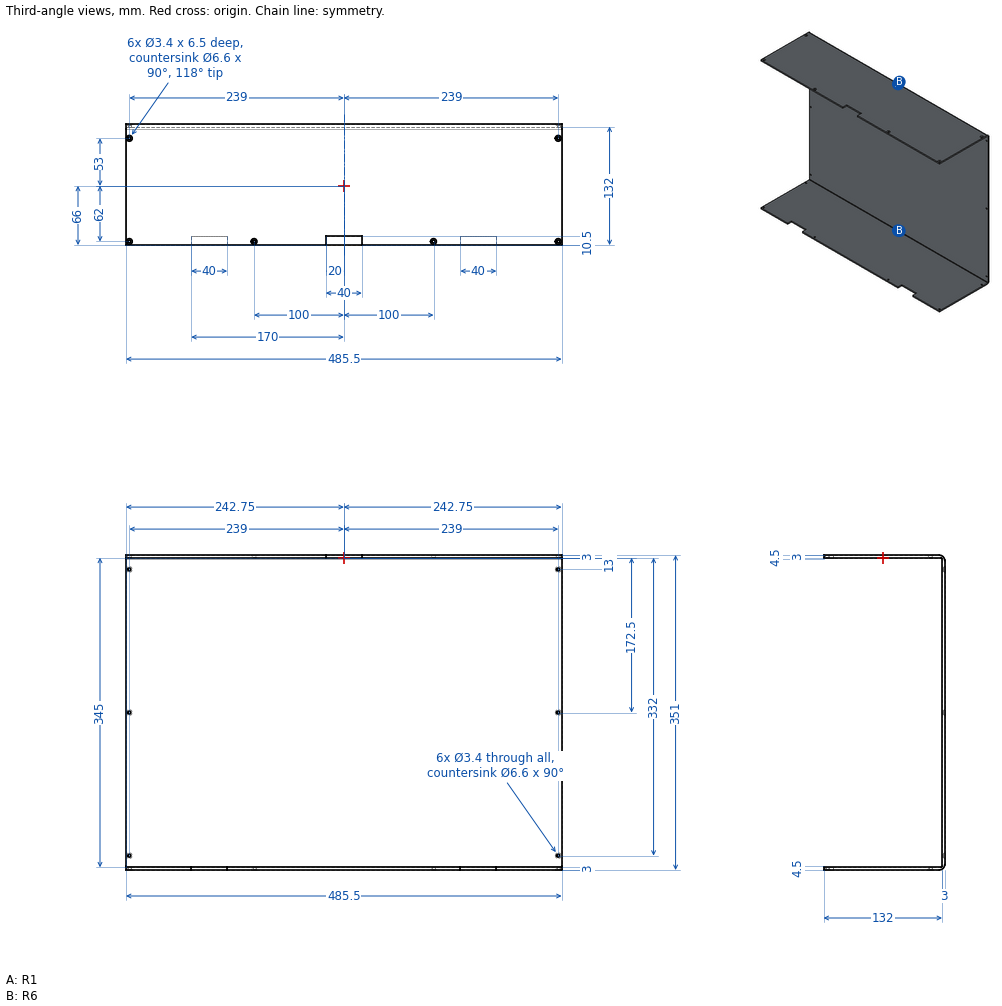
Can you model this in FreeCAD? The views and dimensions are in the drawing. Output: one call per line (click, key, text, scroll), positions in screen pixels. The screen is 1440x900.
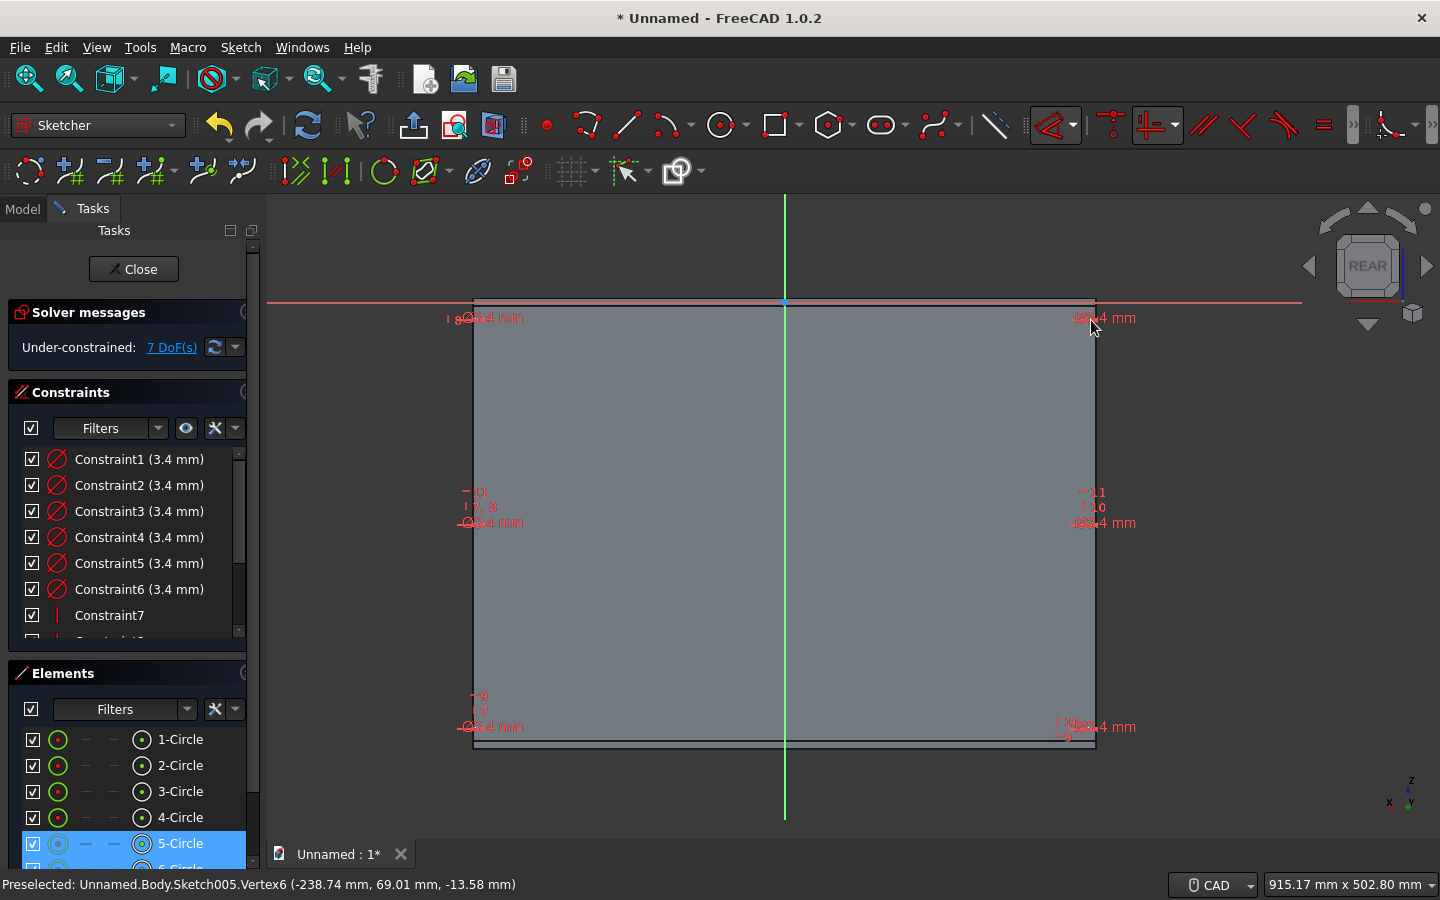
click(1178, 126)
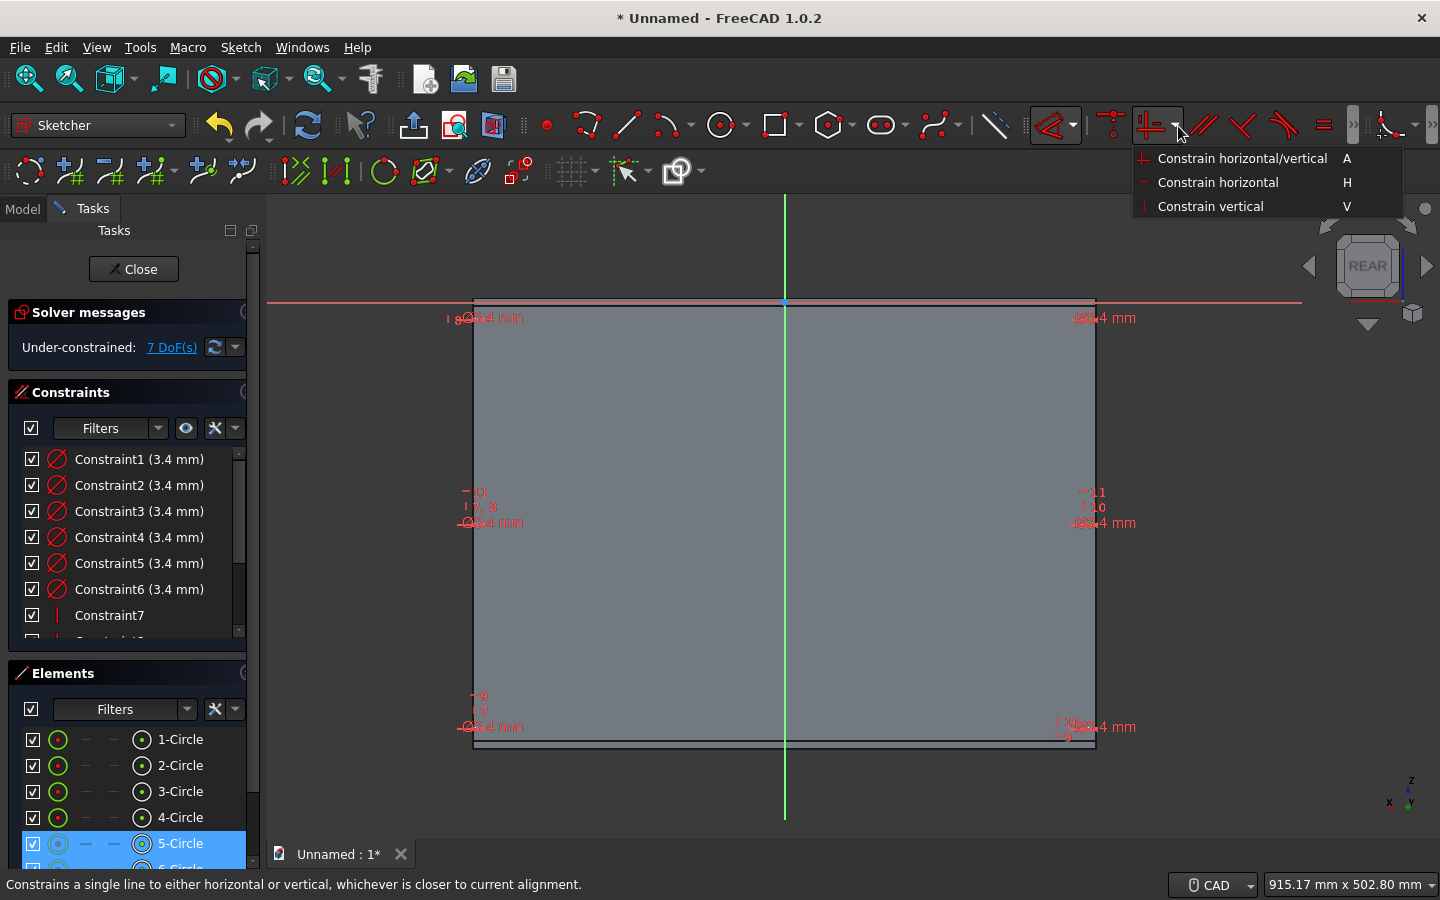
click(1268, 206)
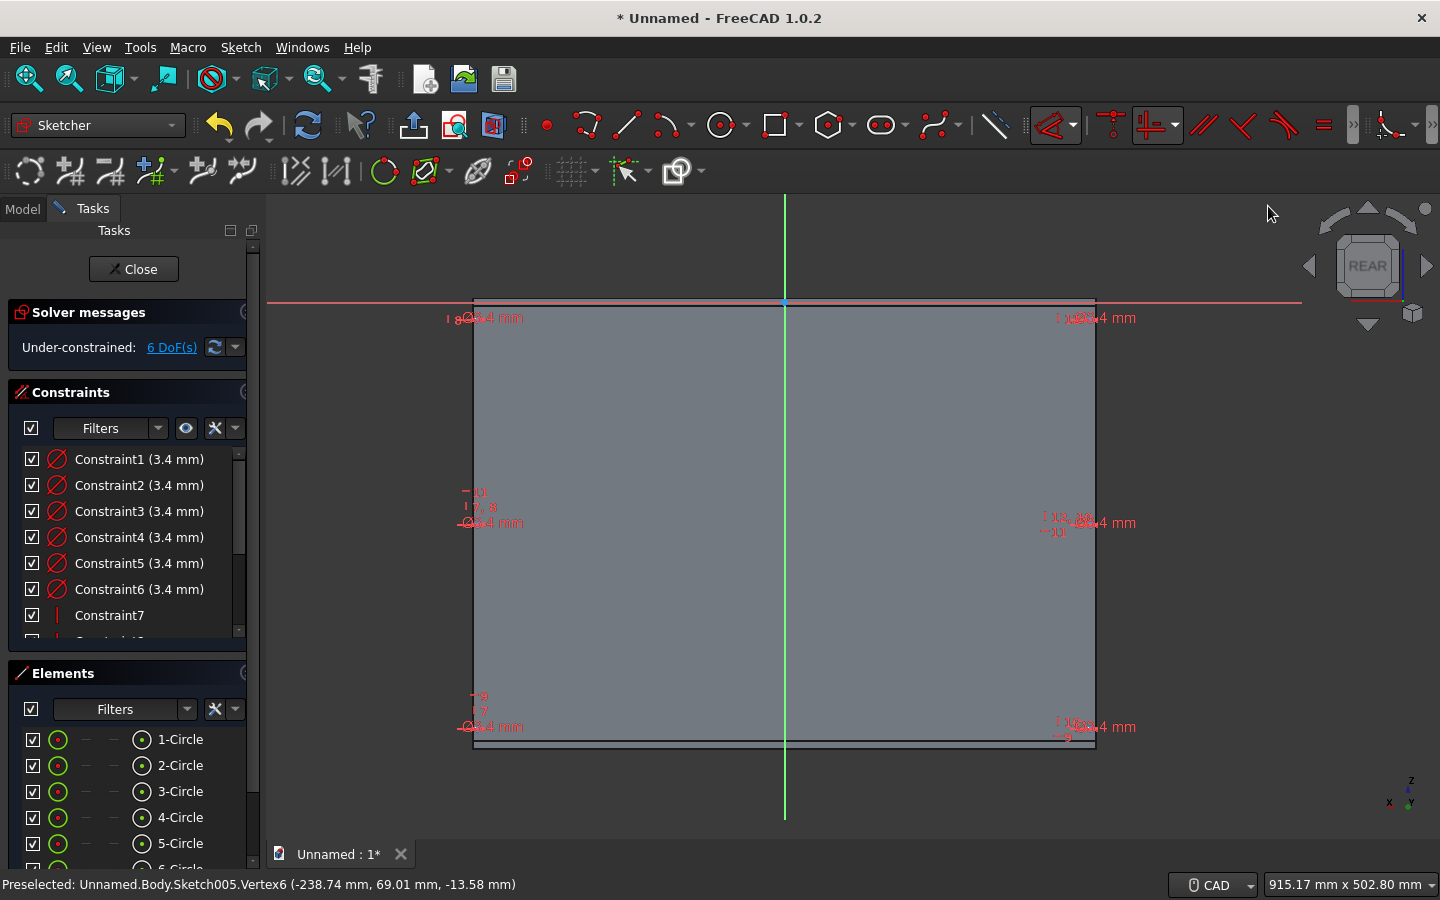
click(478, 320)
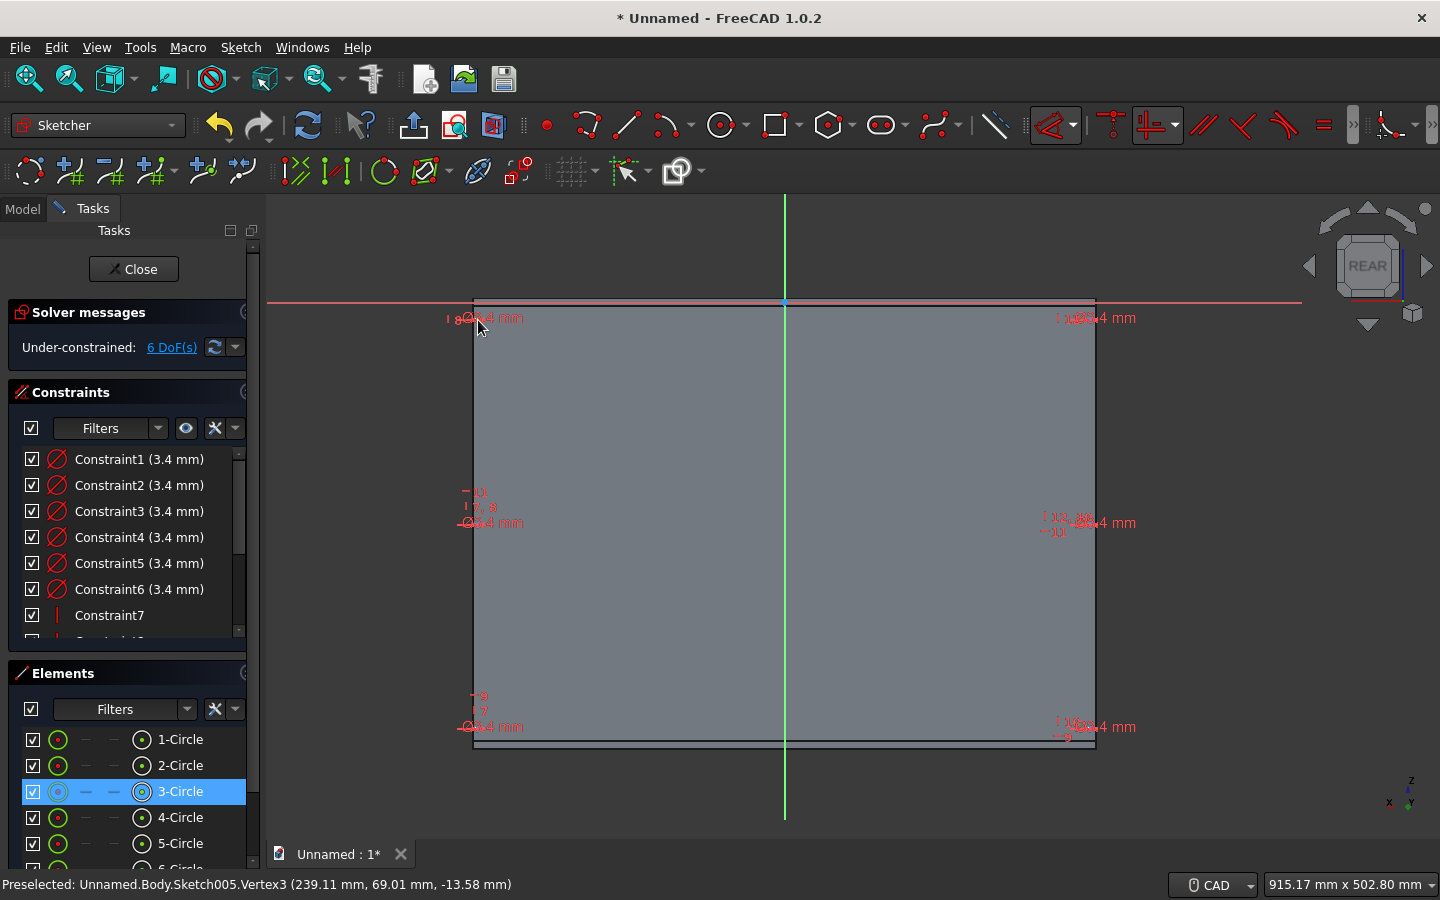
click(1091, 320)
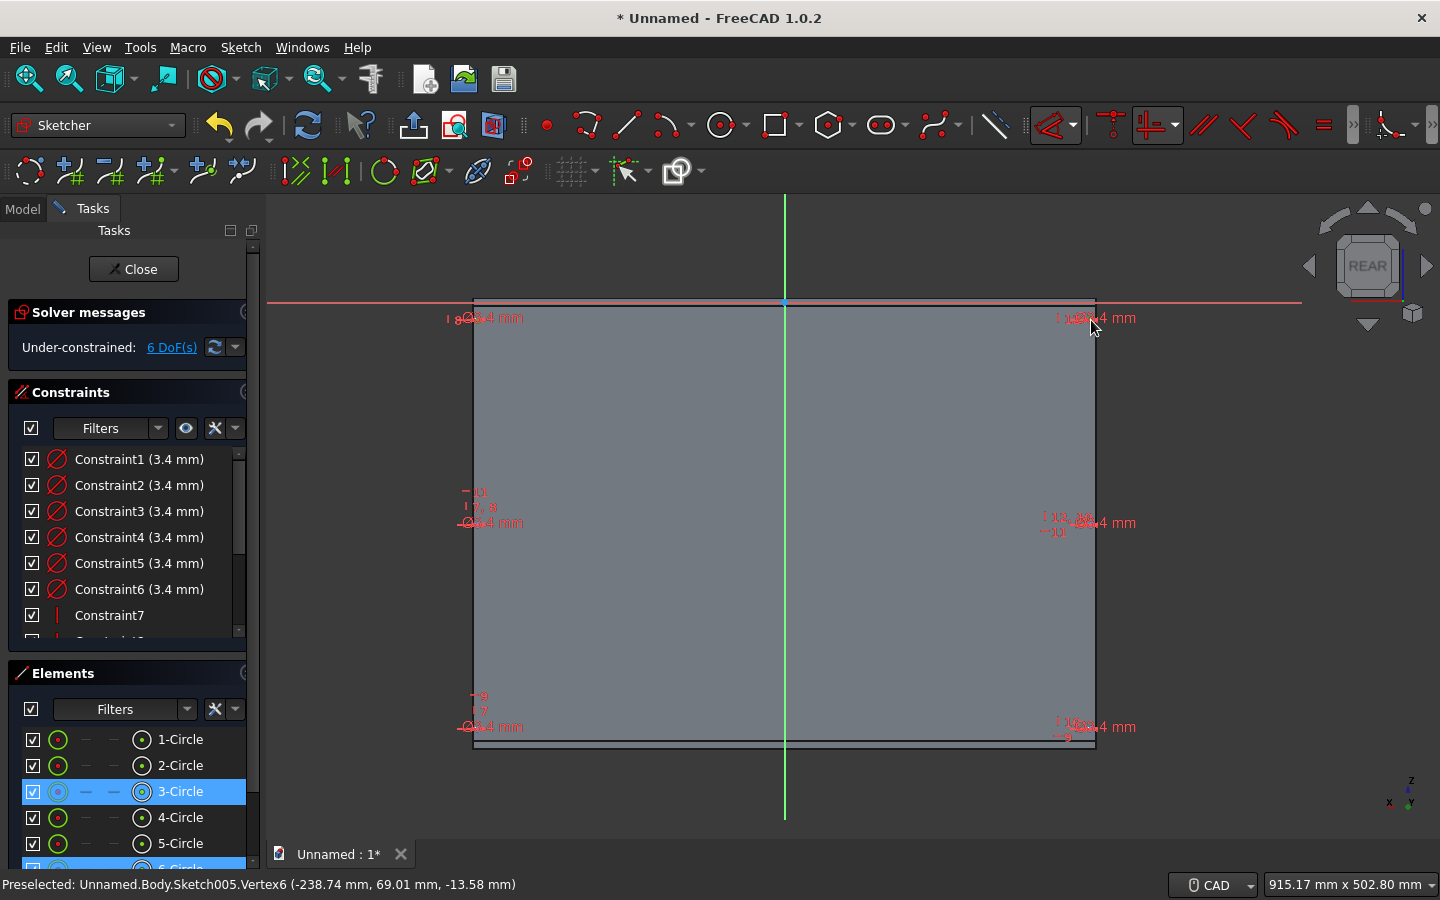
key(h)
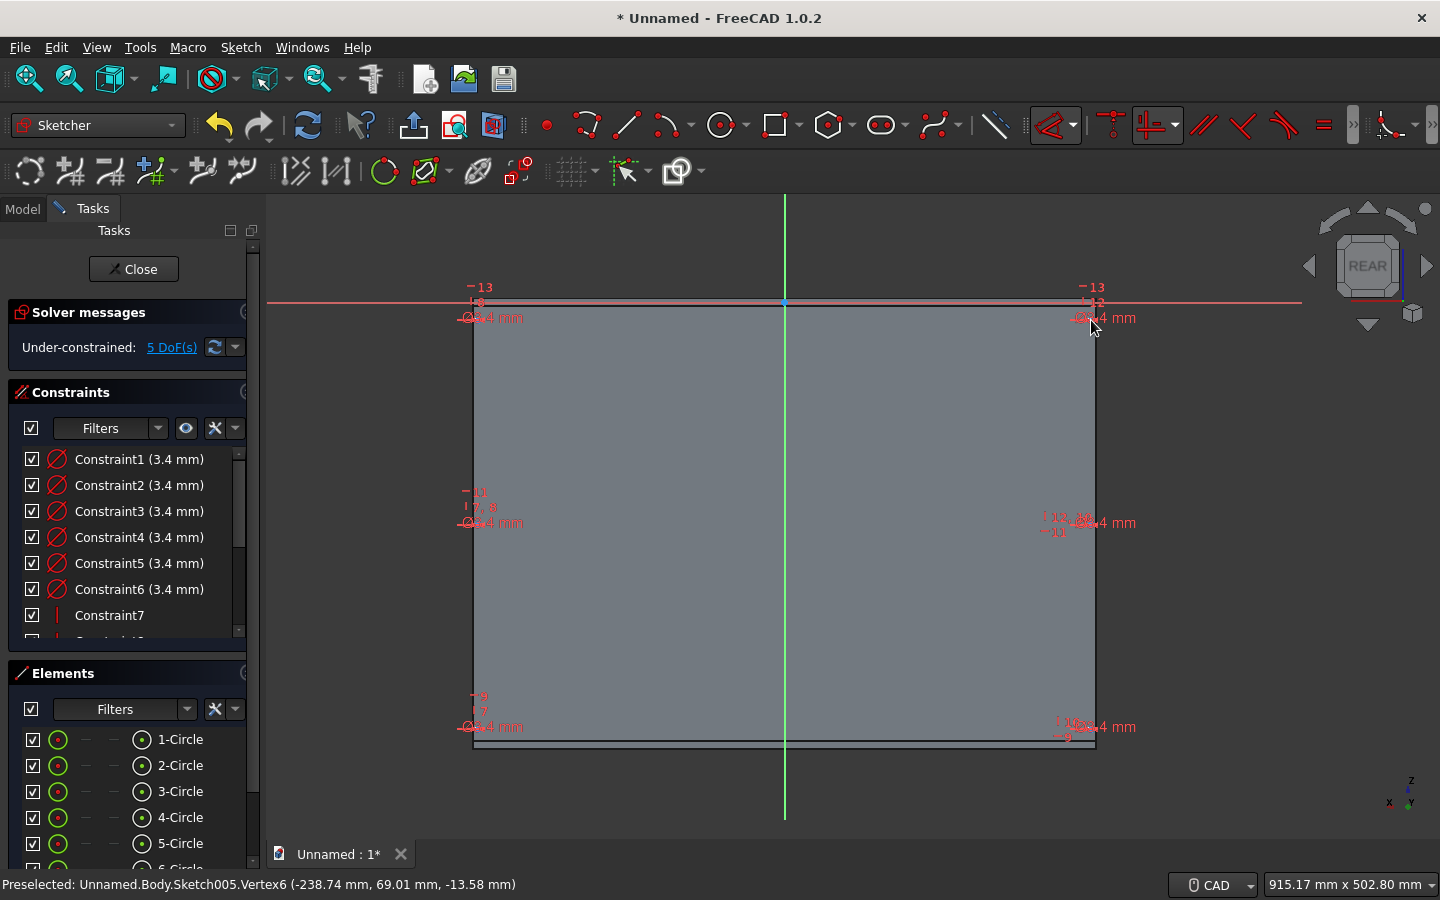
scroll(478, 320, up, 5)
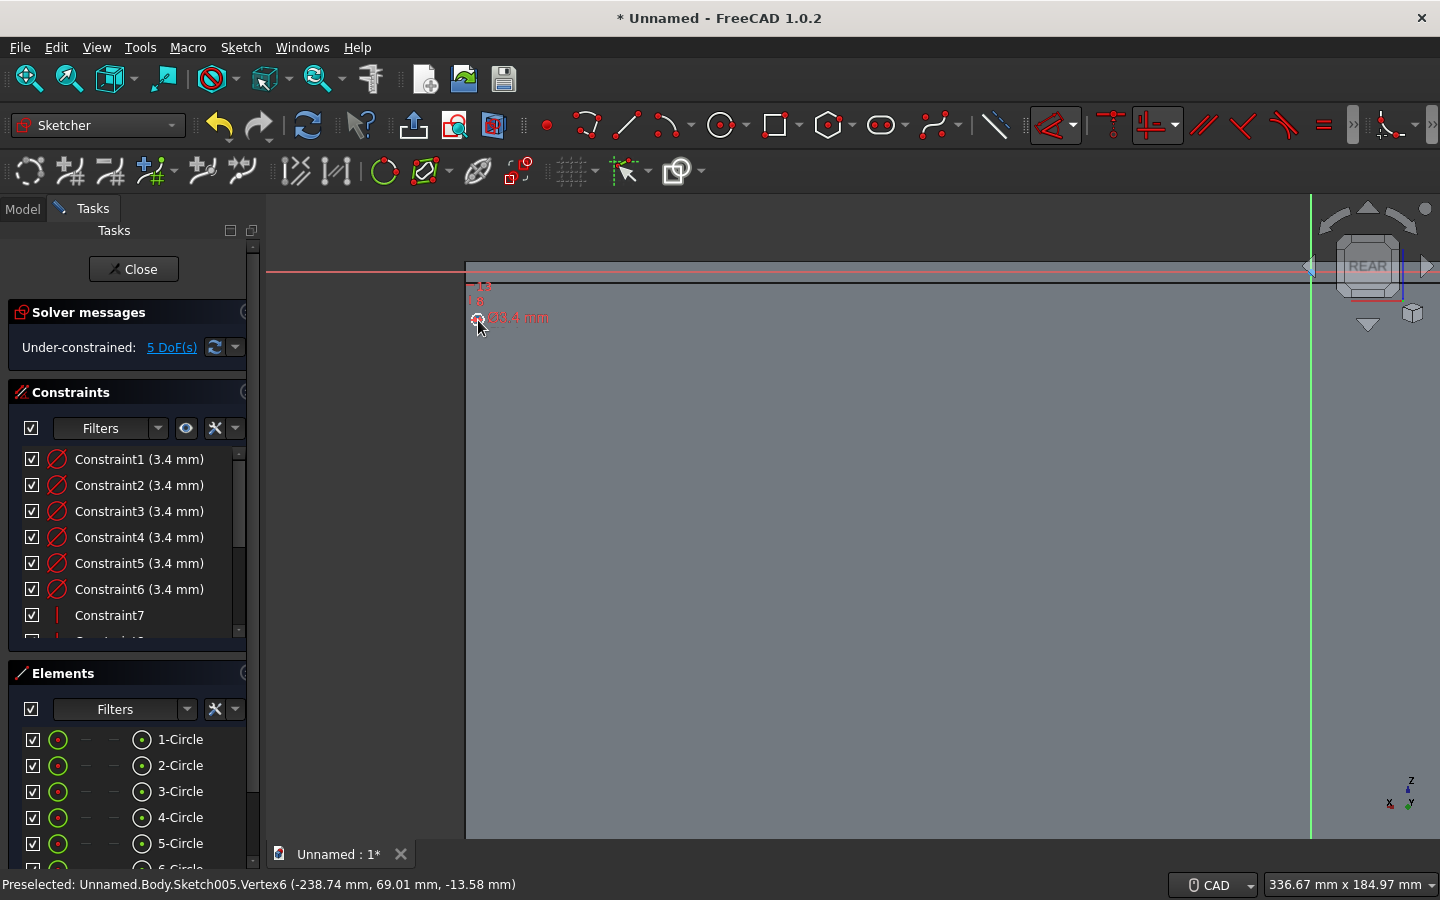
click(478, 320)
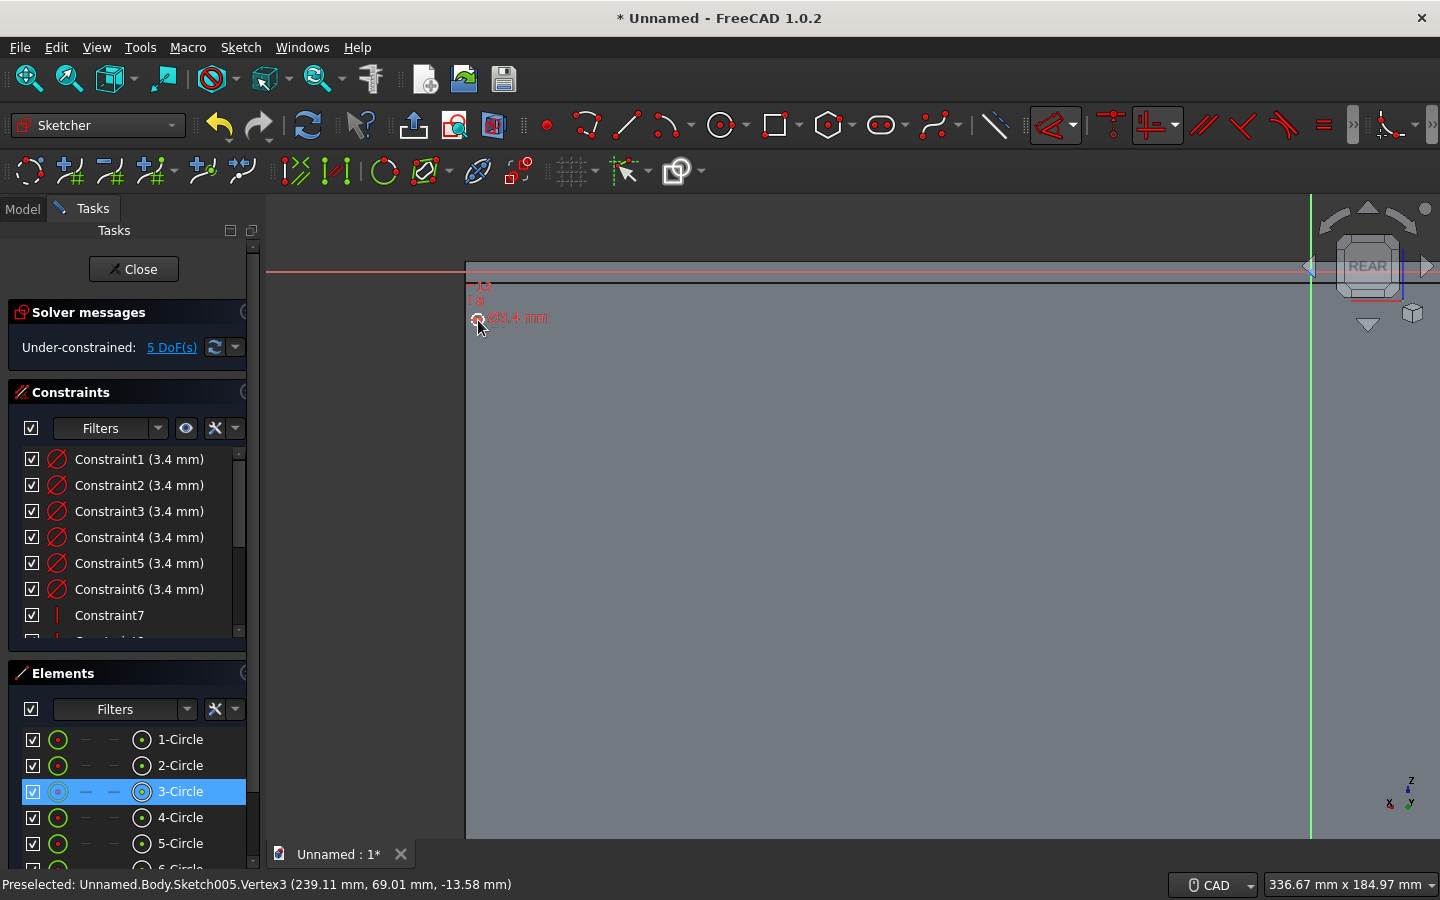
click(1076, 126)